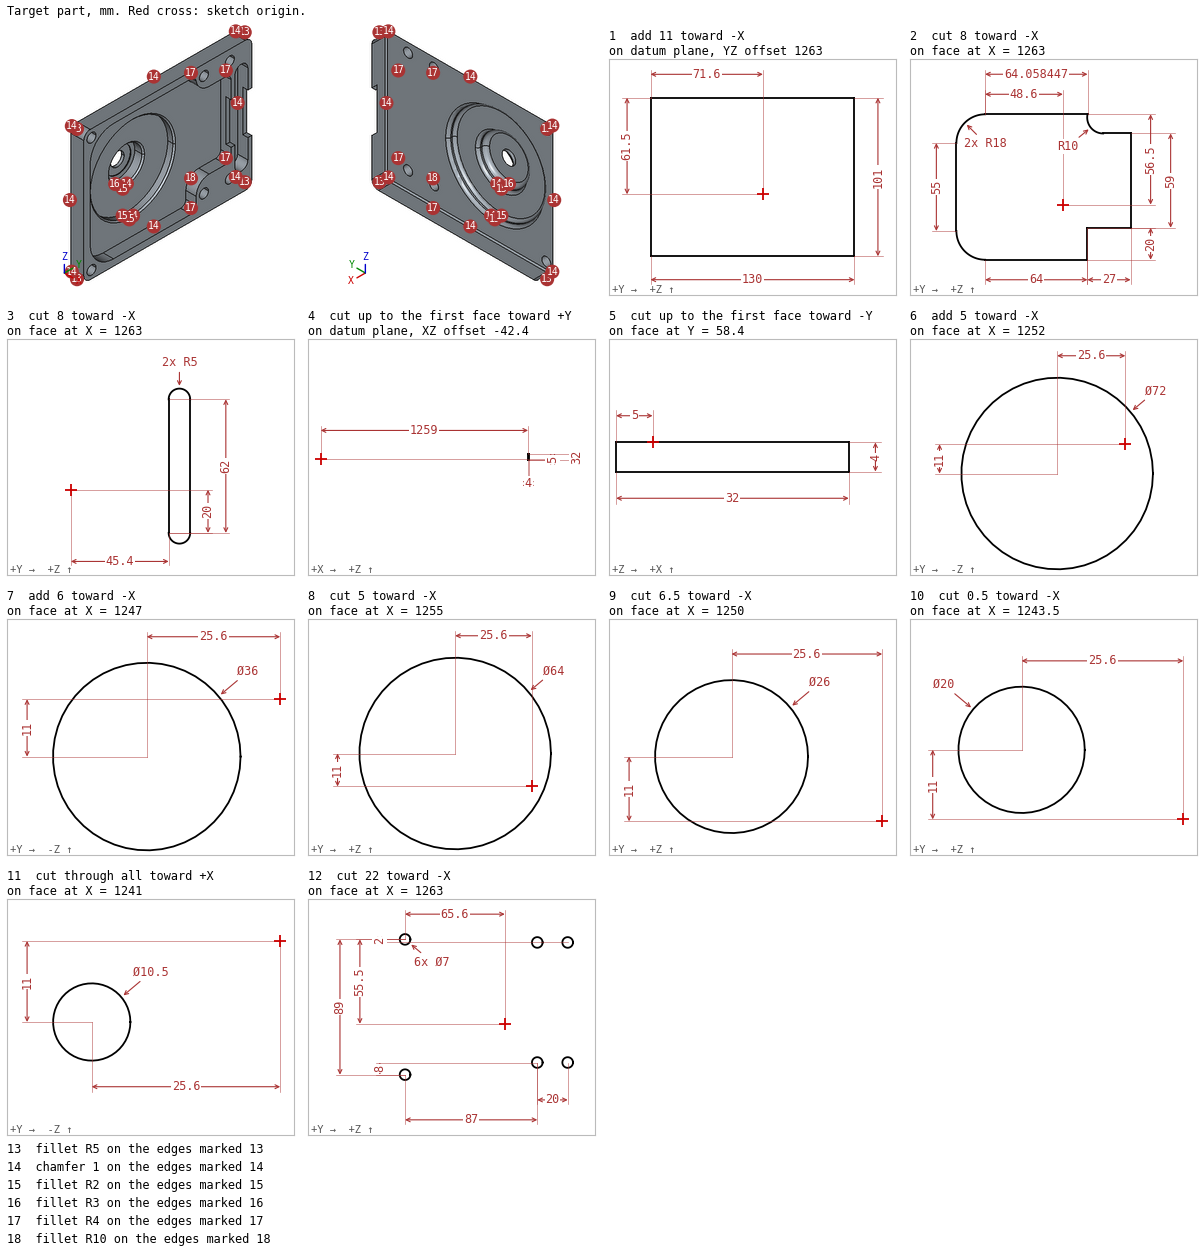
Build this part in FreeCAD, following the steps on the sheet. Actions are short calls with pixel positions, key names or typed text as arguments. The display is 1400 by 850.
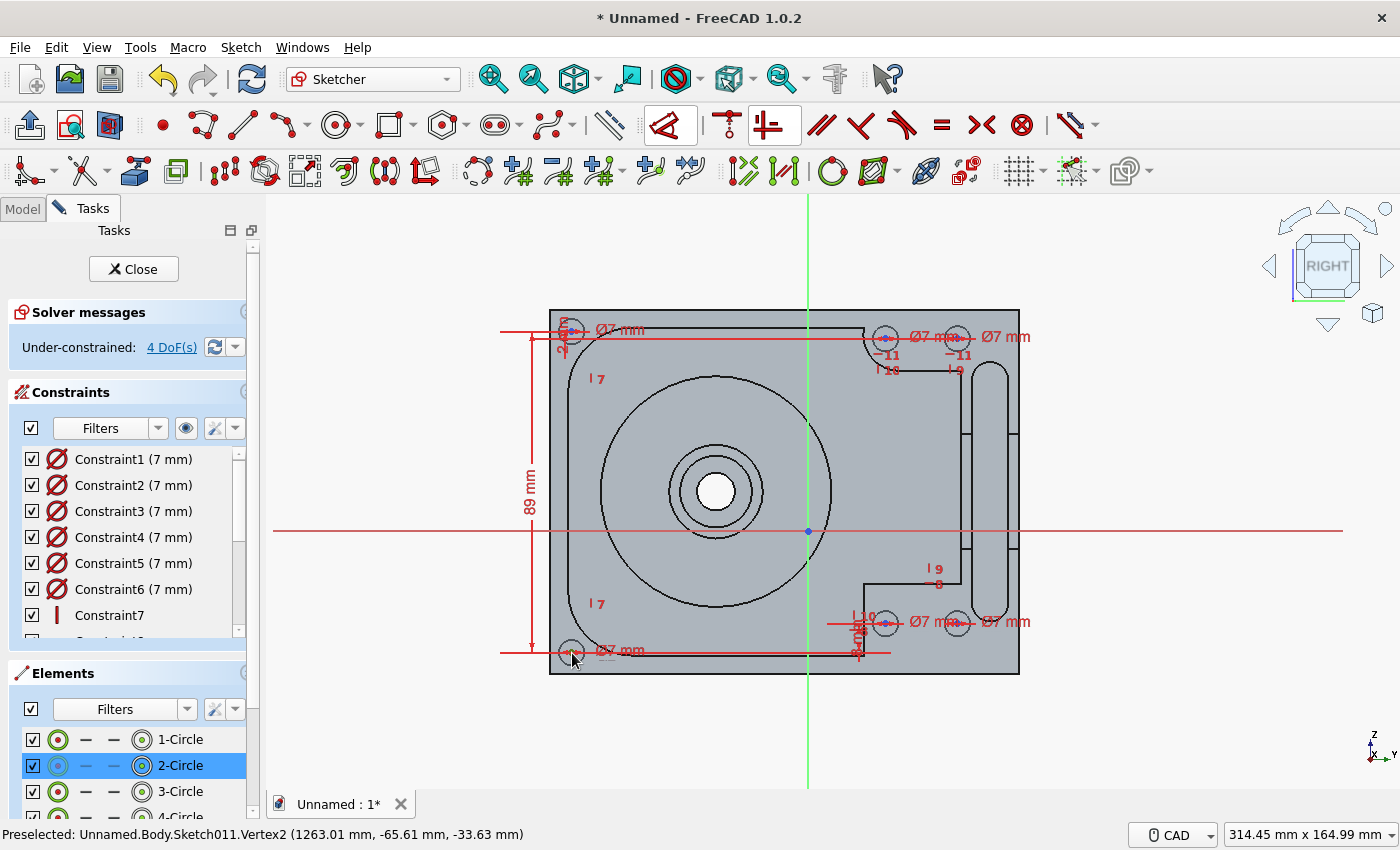
click(886, 624)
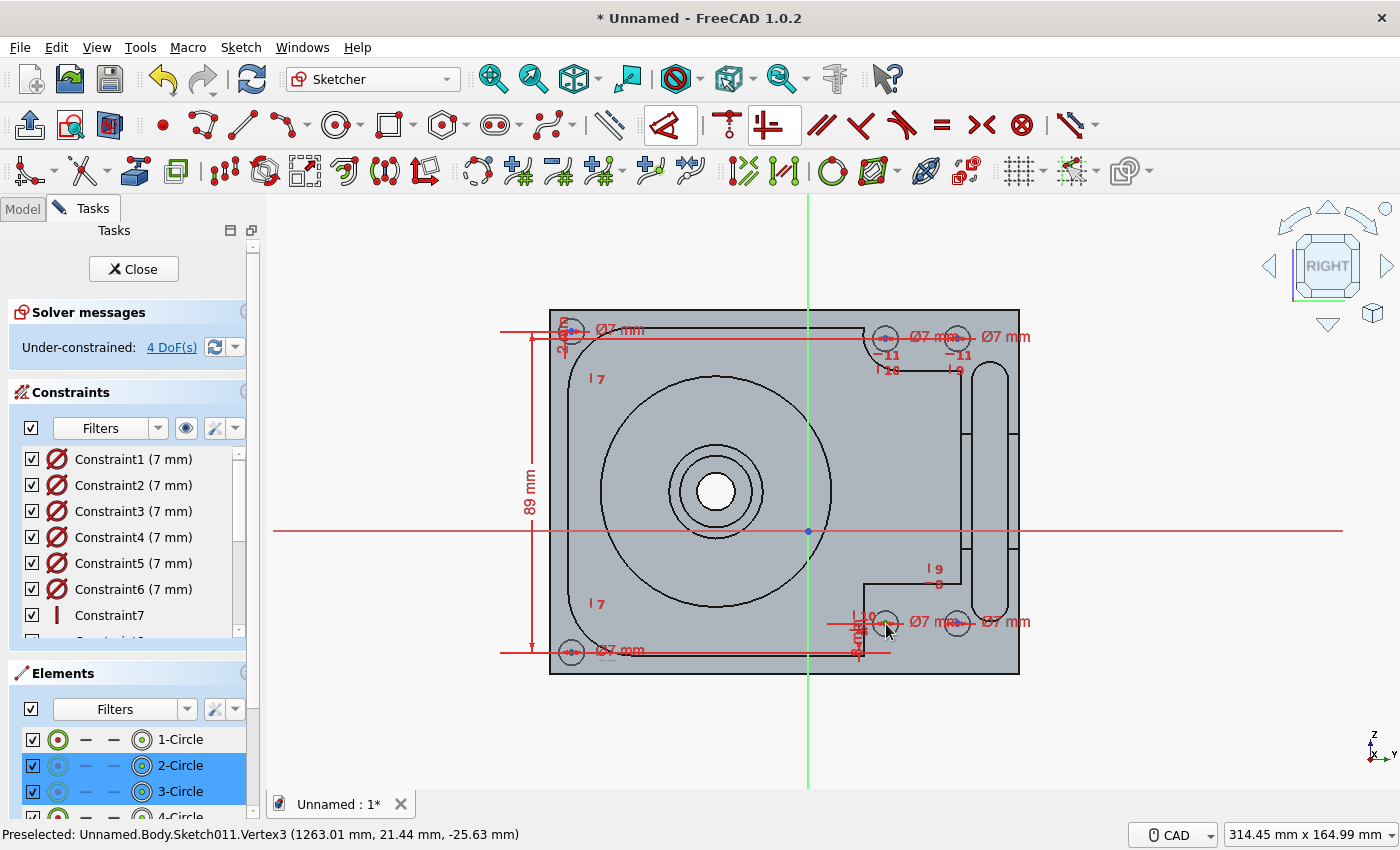
key(l)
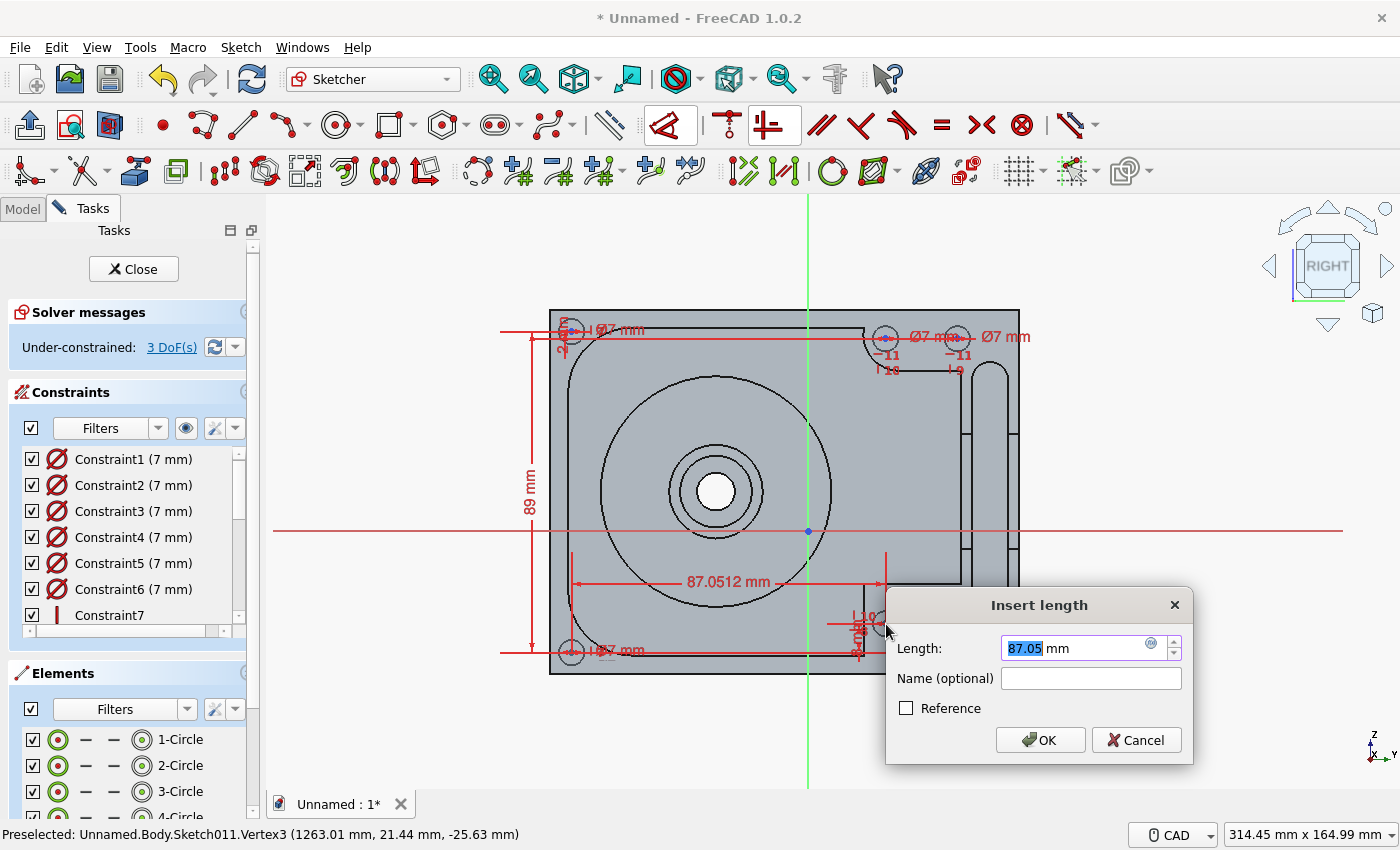
text(87)
key(Return)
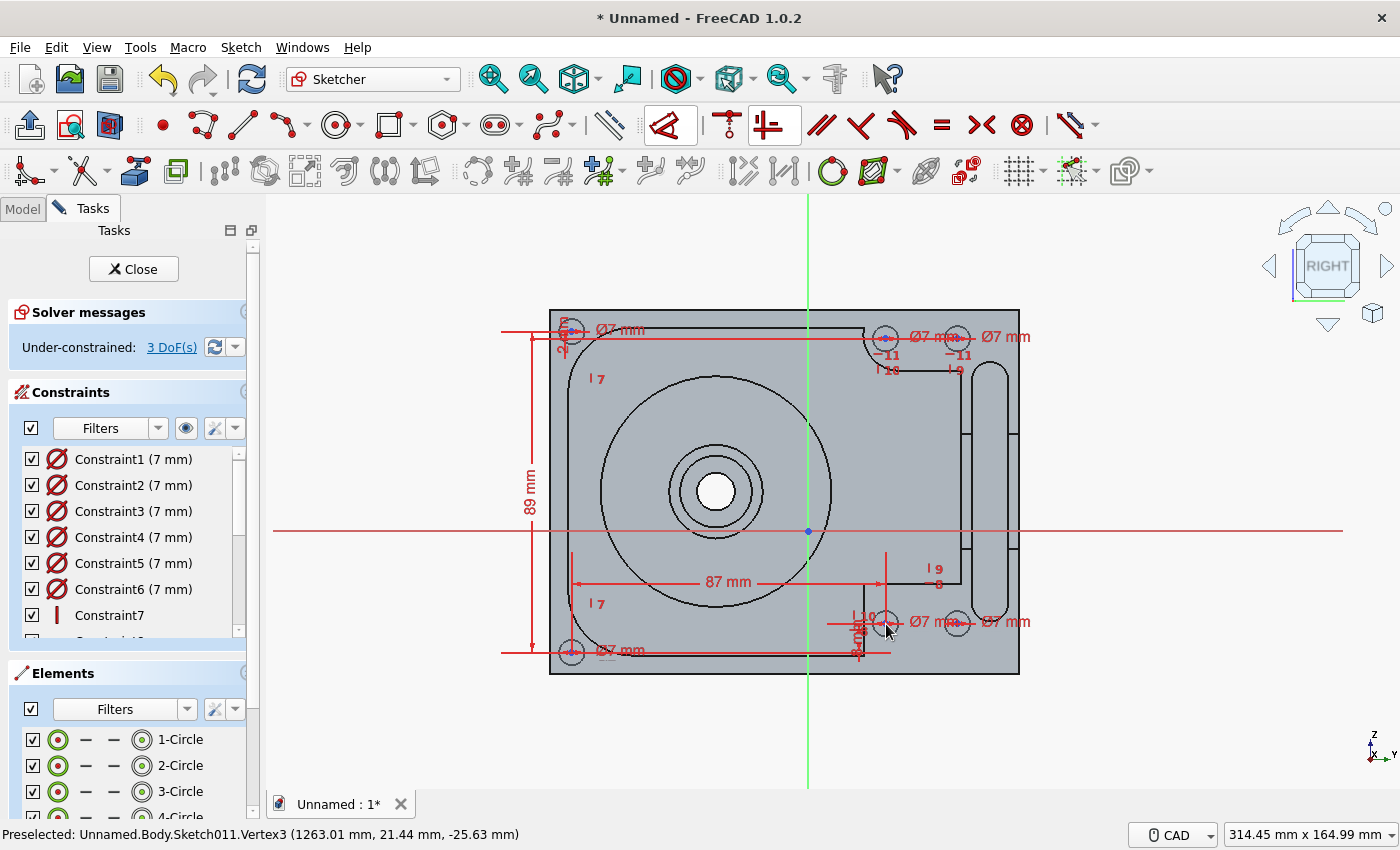
click(886, 624)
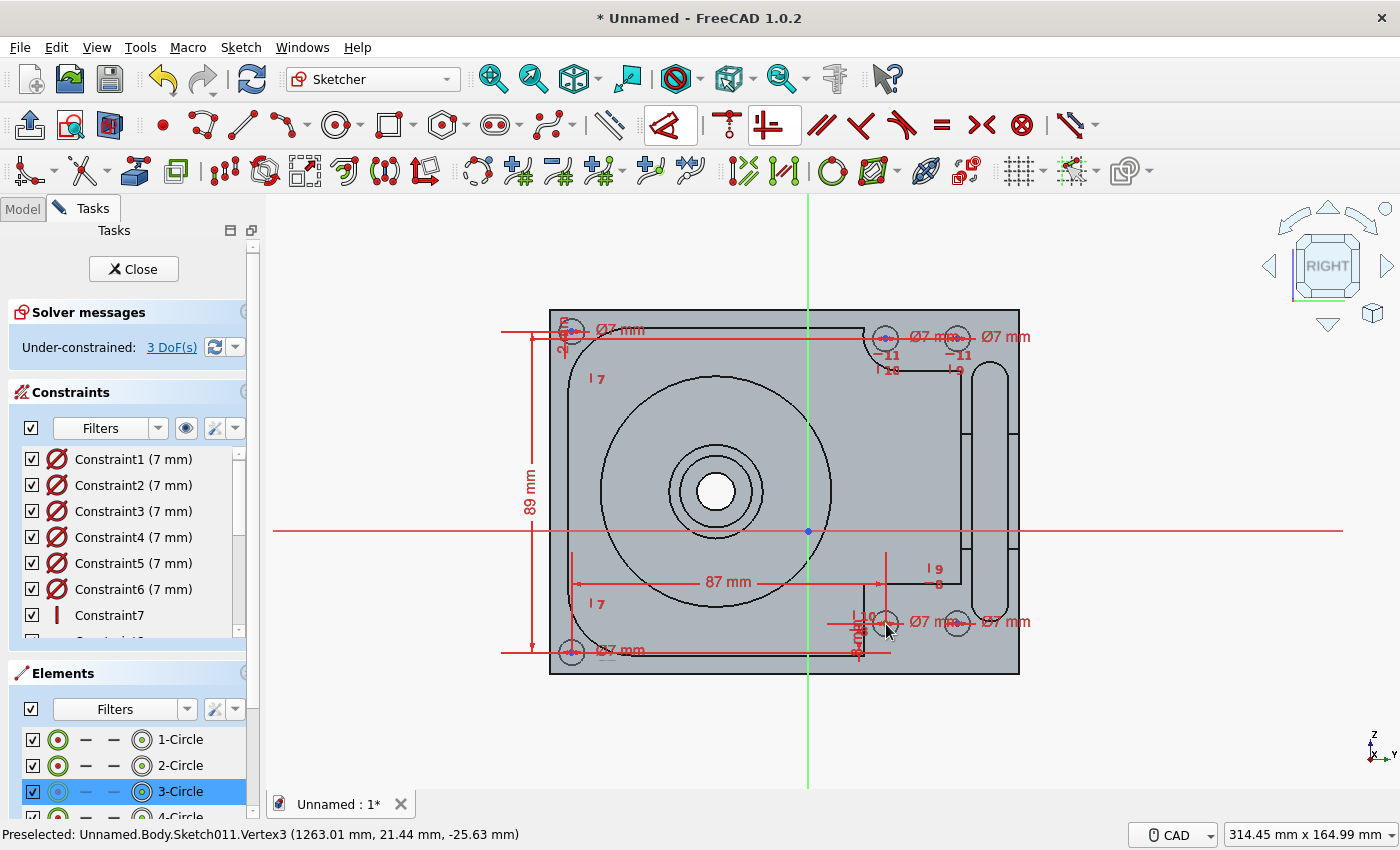
click(957, 624)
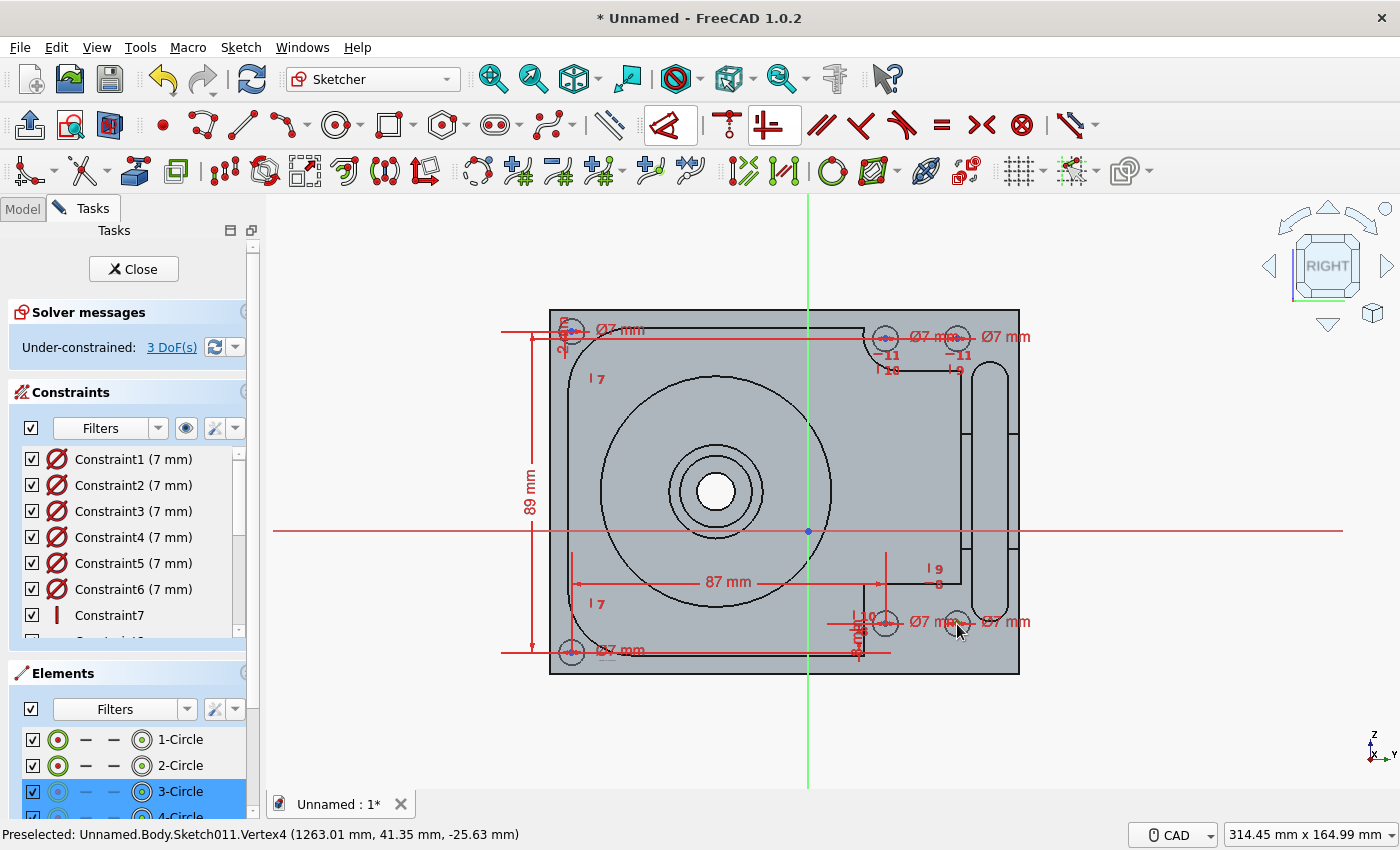
key(l)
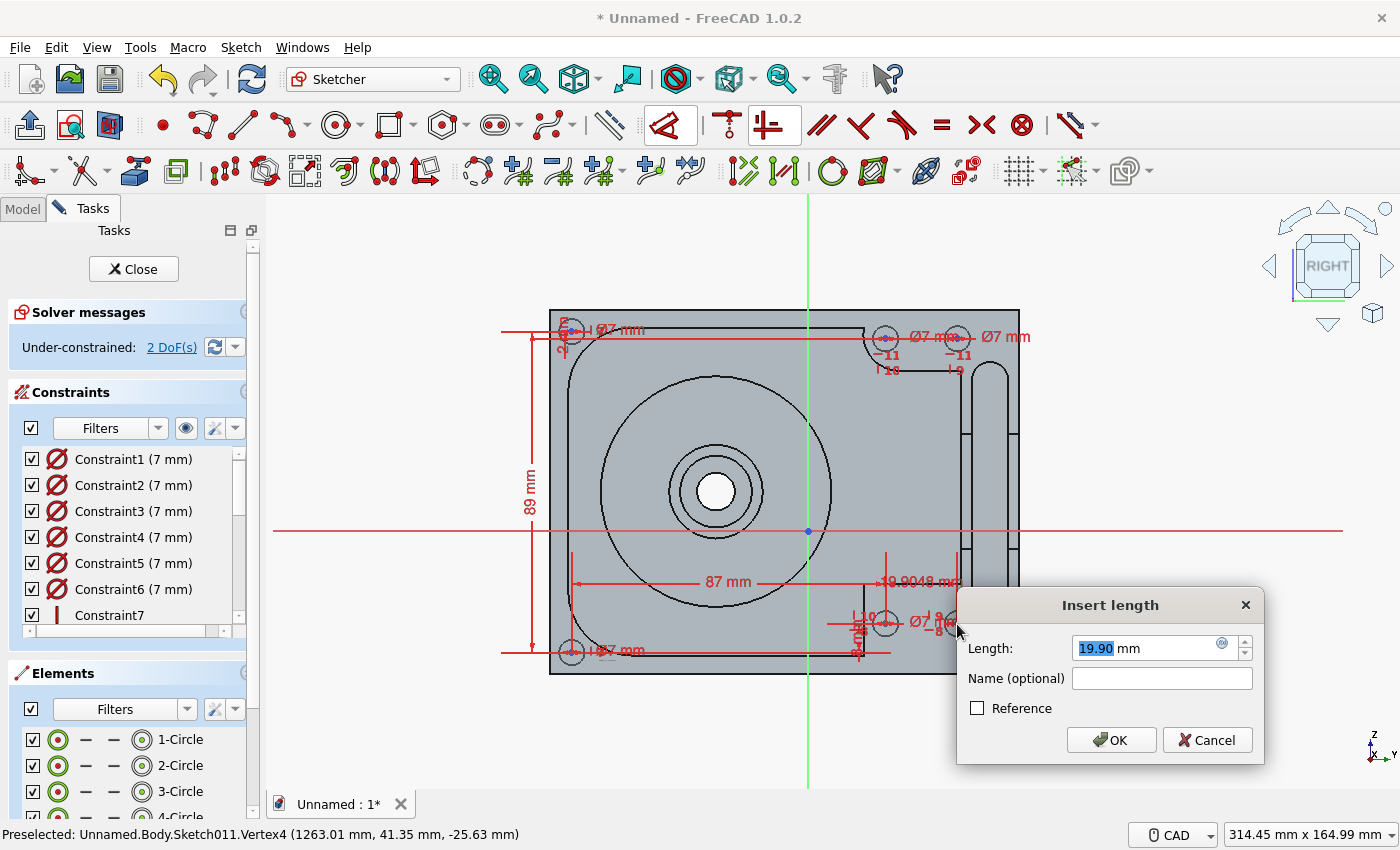
text(20)
key(Return)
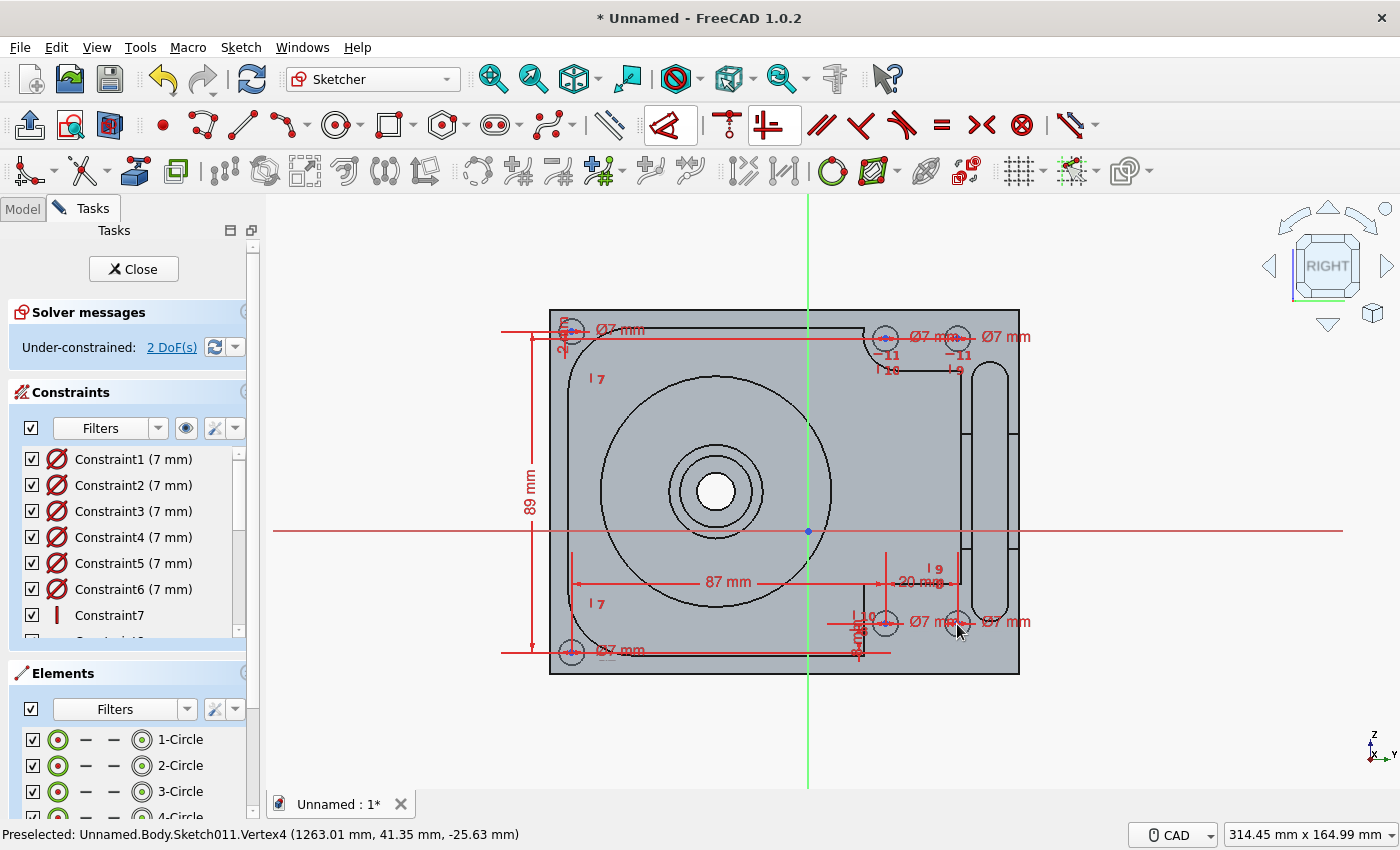
click(572, 332)